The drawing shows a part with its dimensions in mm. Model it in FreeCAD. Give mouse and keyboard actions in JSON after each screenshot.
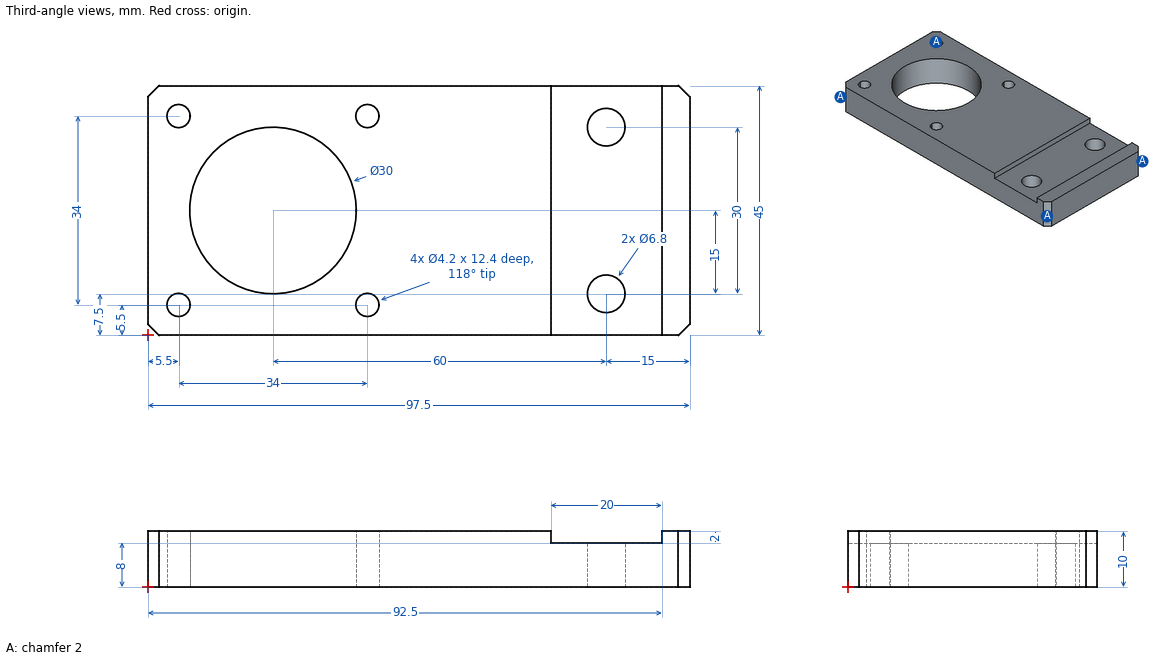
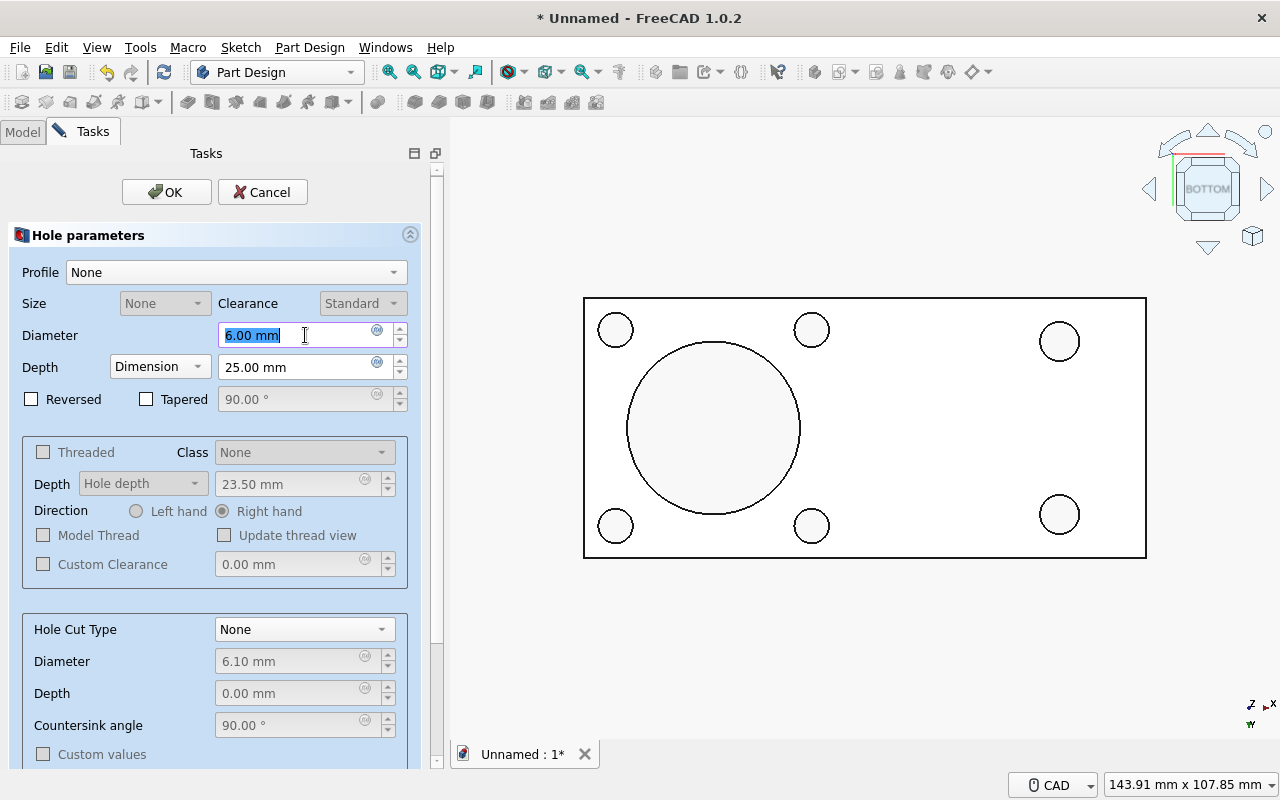
{"action": "type", "text": "4.2"}
{"action": "key", "text": "Tab"}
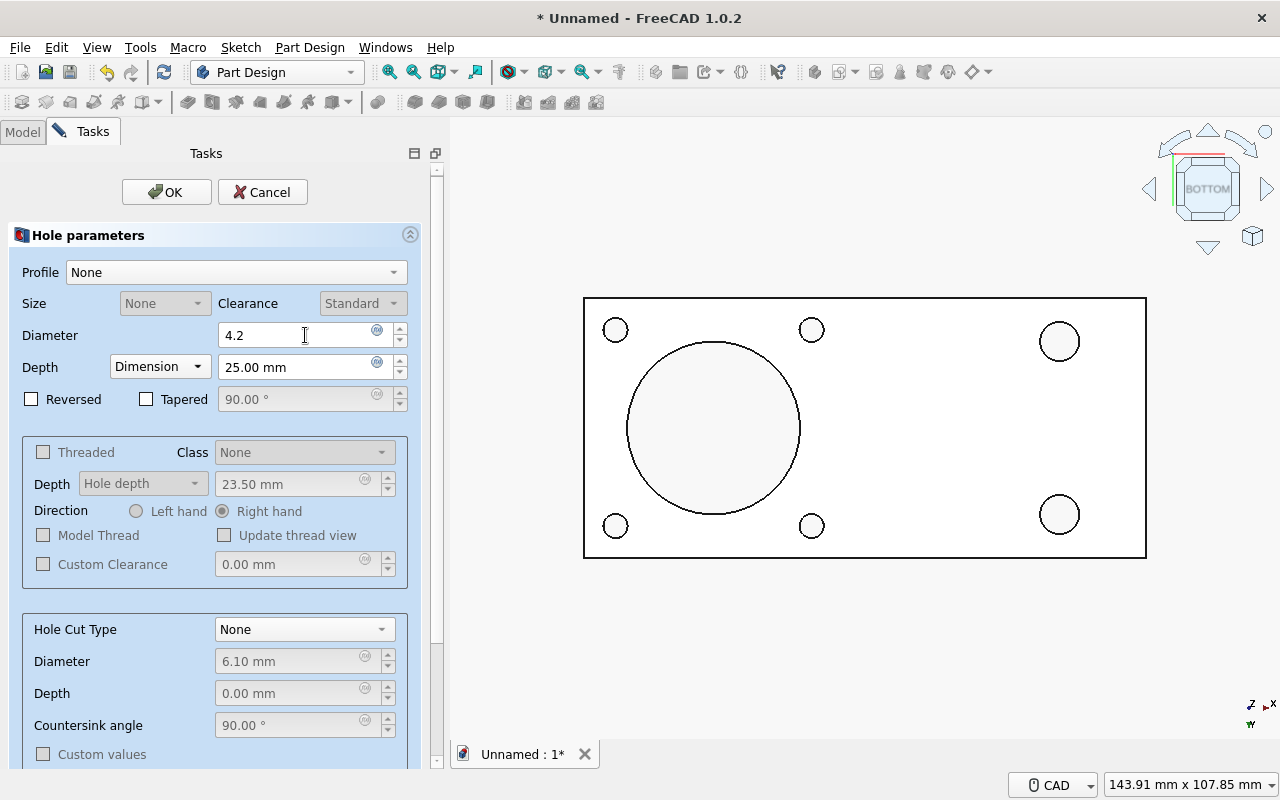
{"action": "triple_click", "coordinate": [305, 367]}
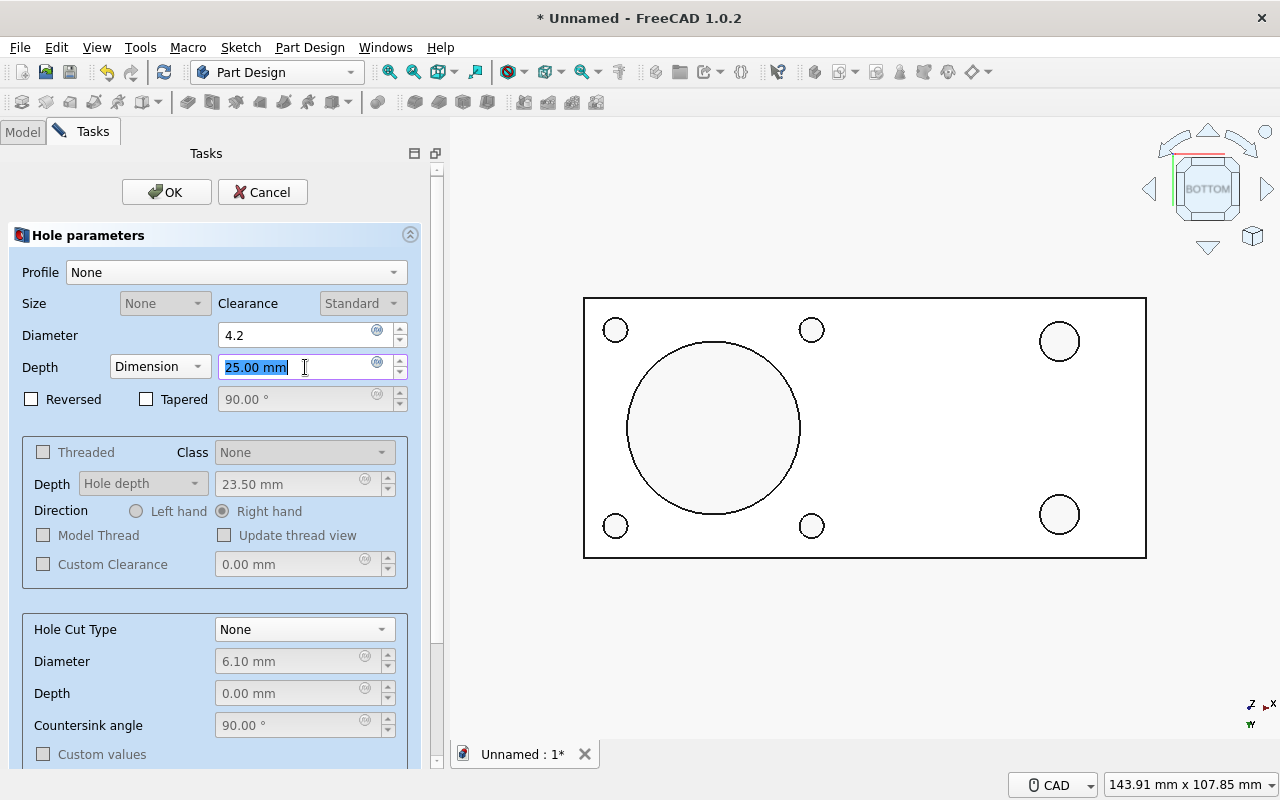
{"action": "type", "text": "12.4"}
{"action": "key", "text": "Tab"}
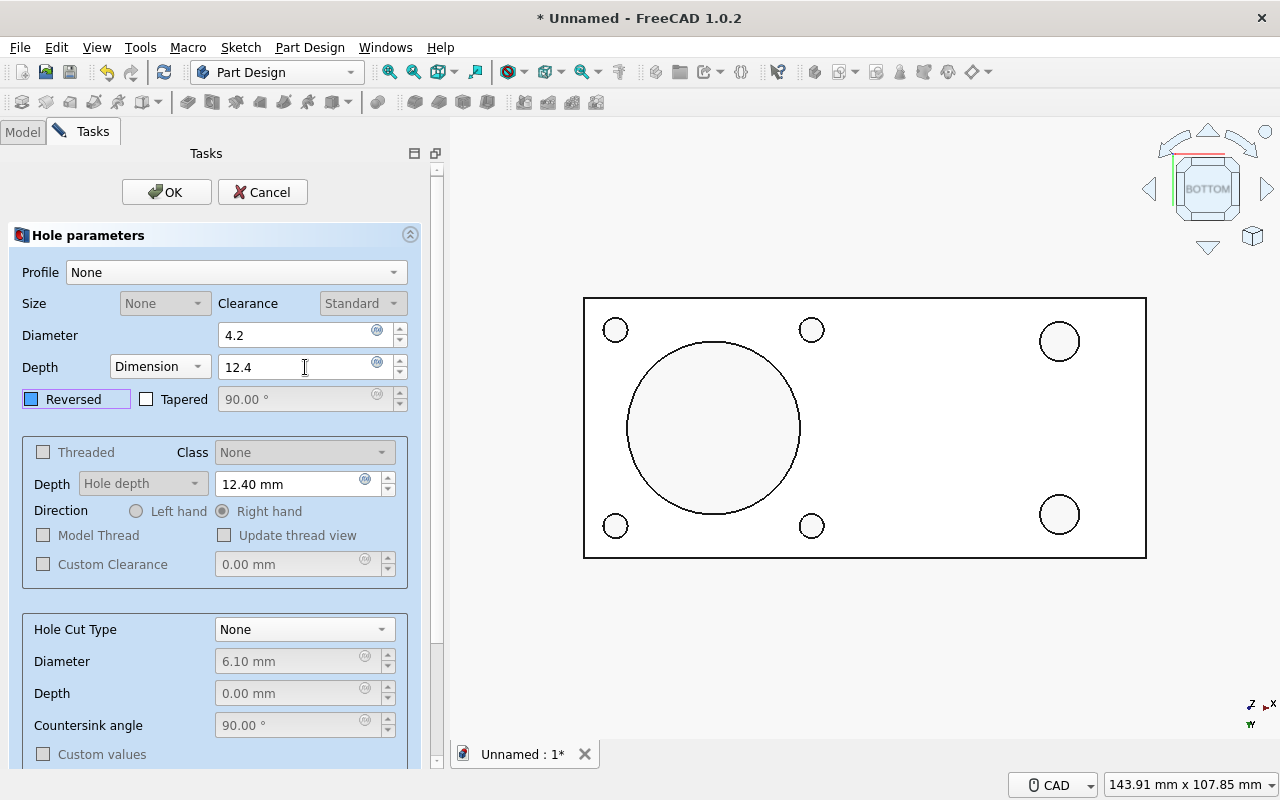
{"action": "left_click", "coordinate": [167, 192]}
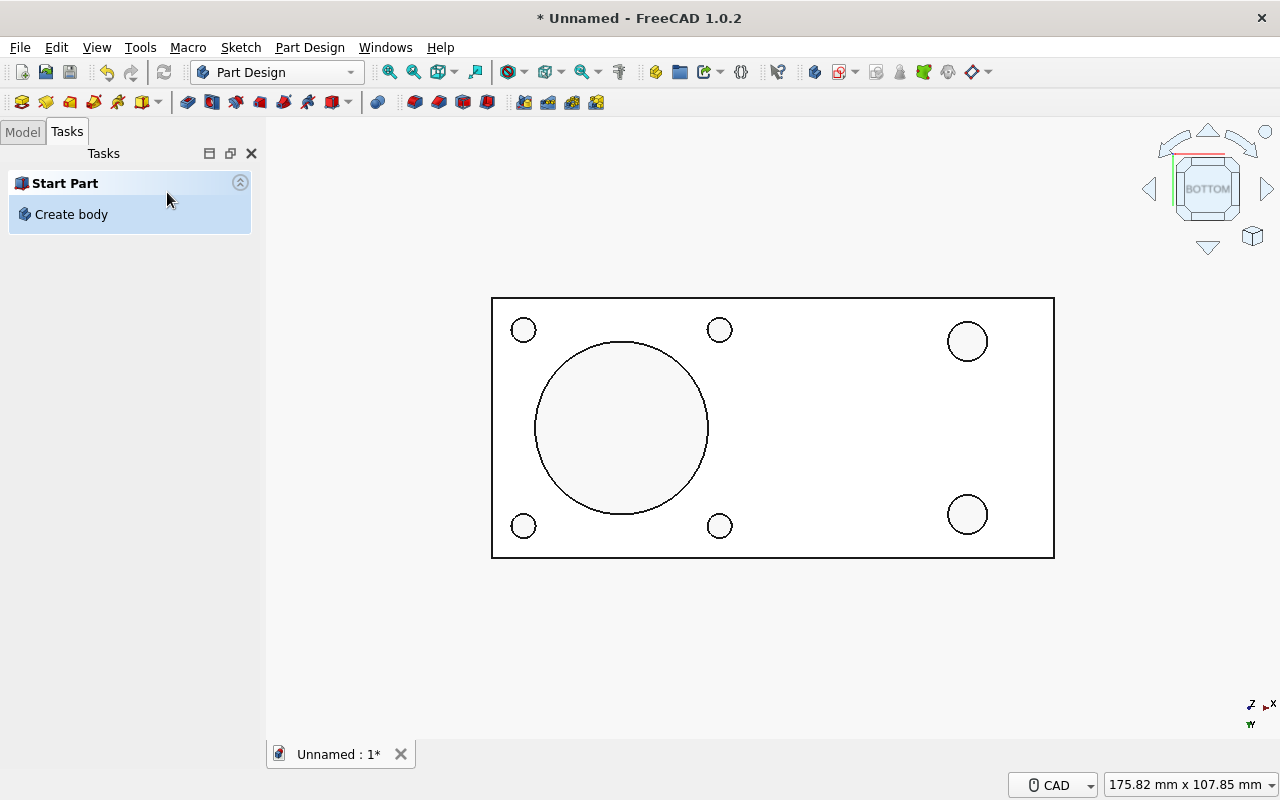
{"action": "key", "text": "0"}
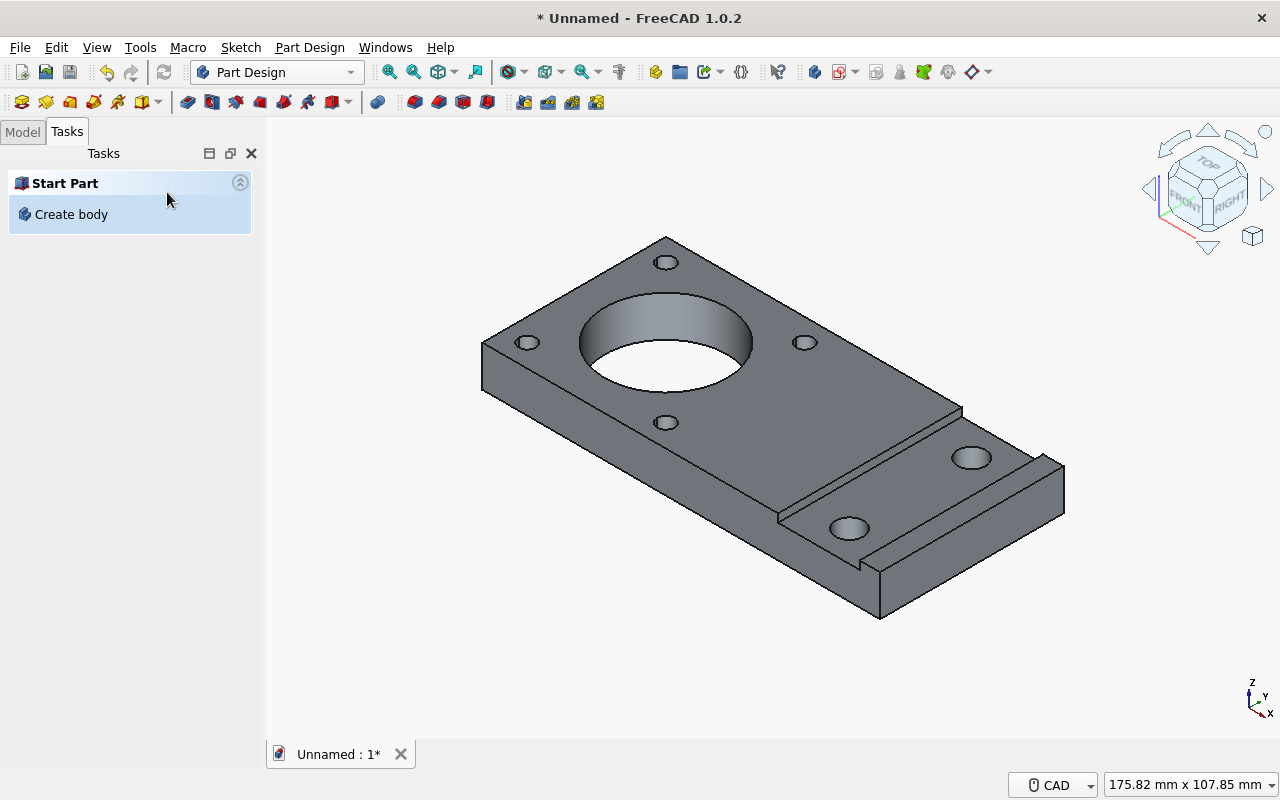
{"action": "left_click", "coordinate": [880, 595]}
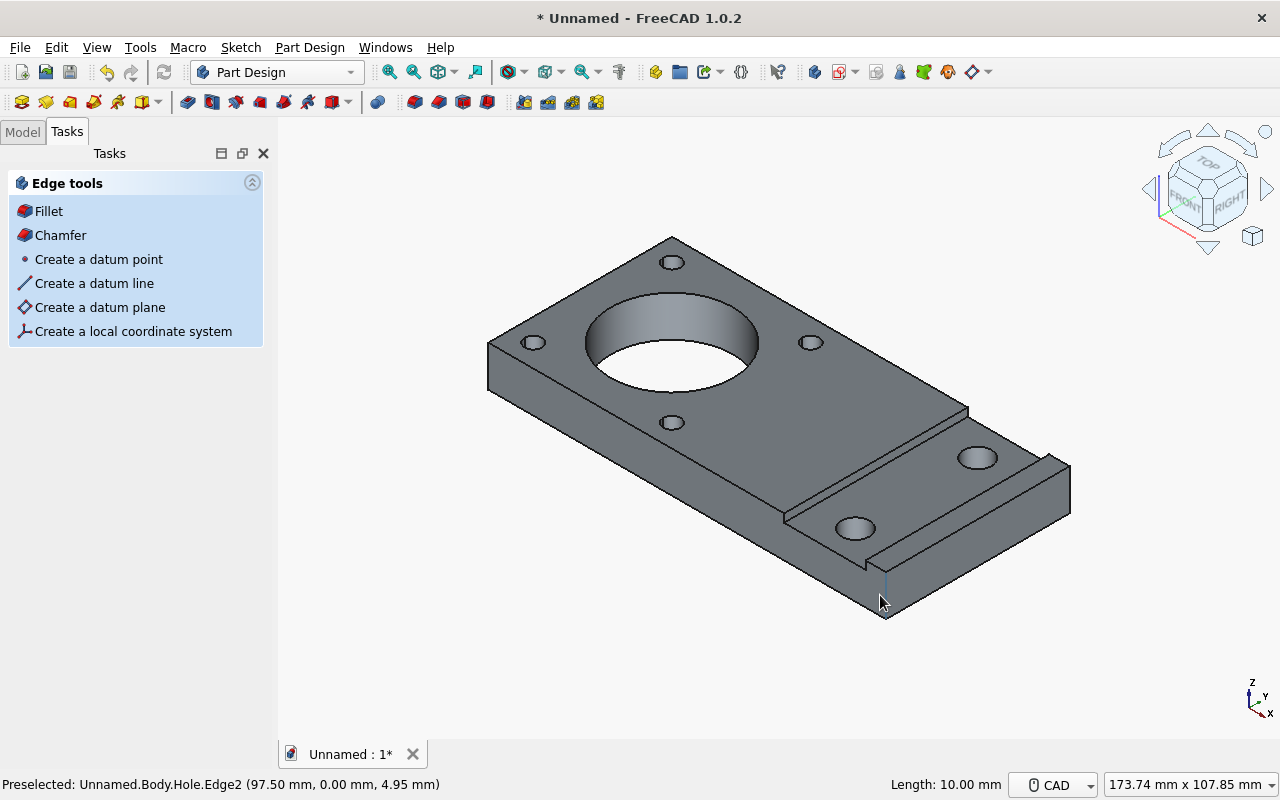
{"action": "key", "text": "2"}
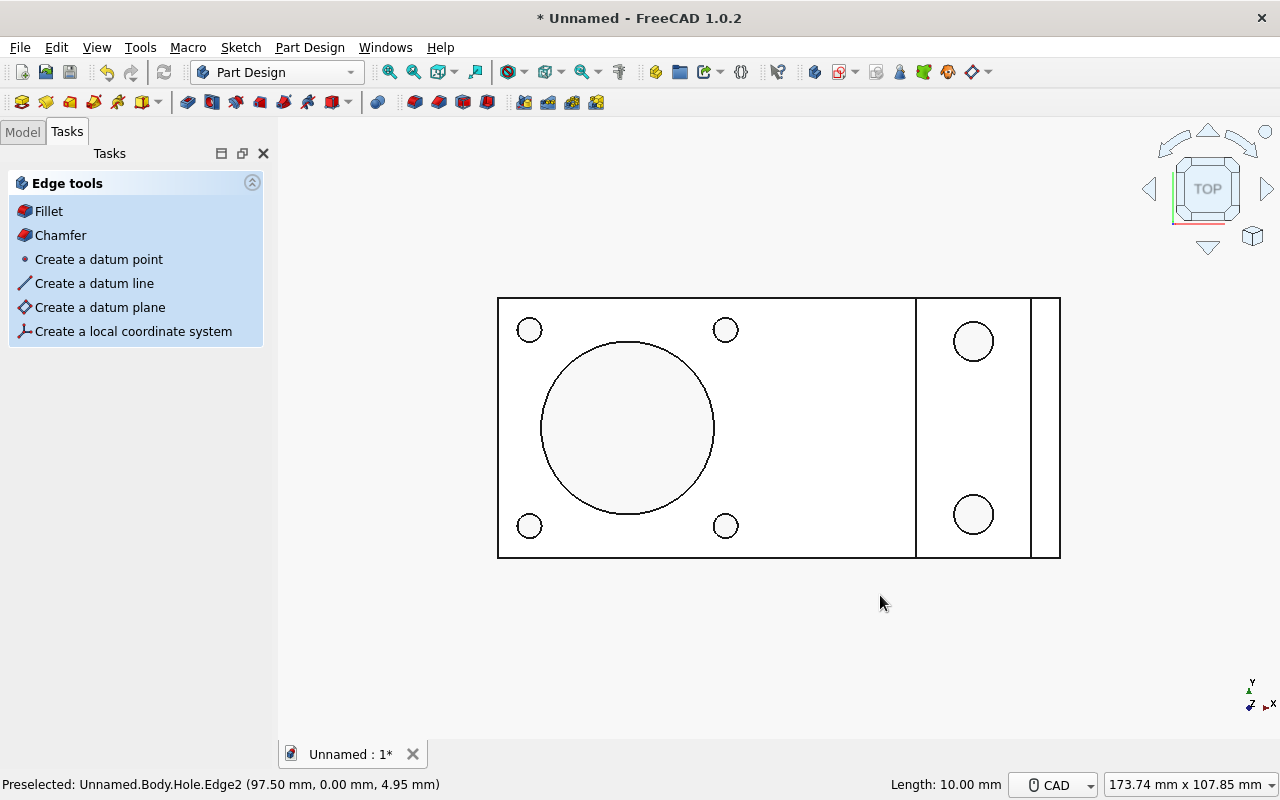
{"action": "key", "text": "1"}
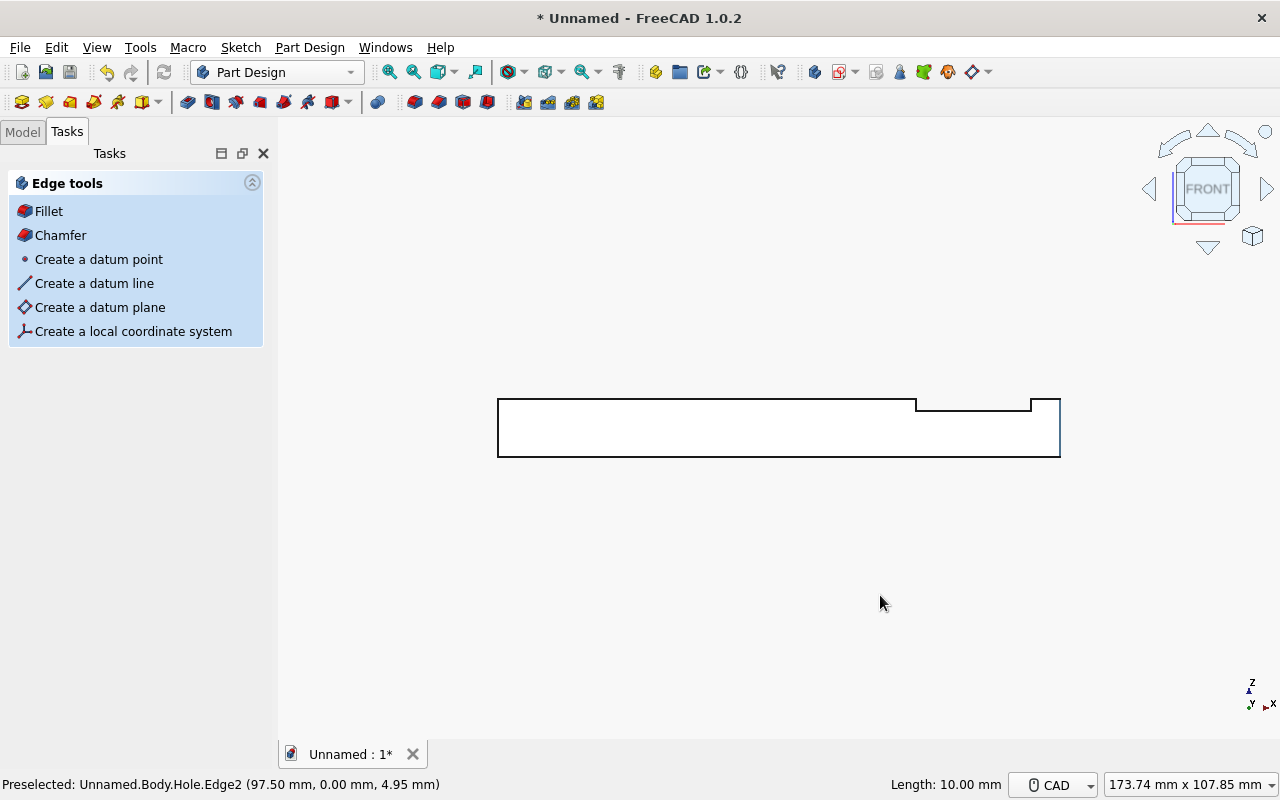
{"action": "left_click", "coordinate": [498, 427], "text": "ctrl"}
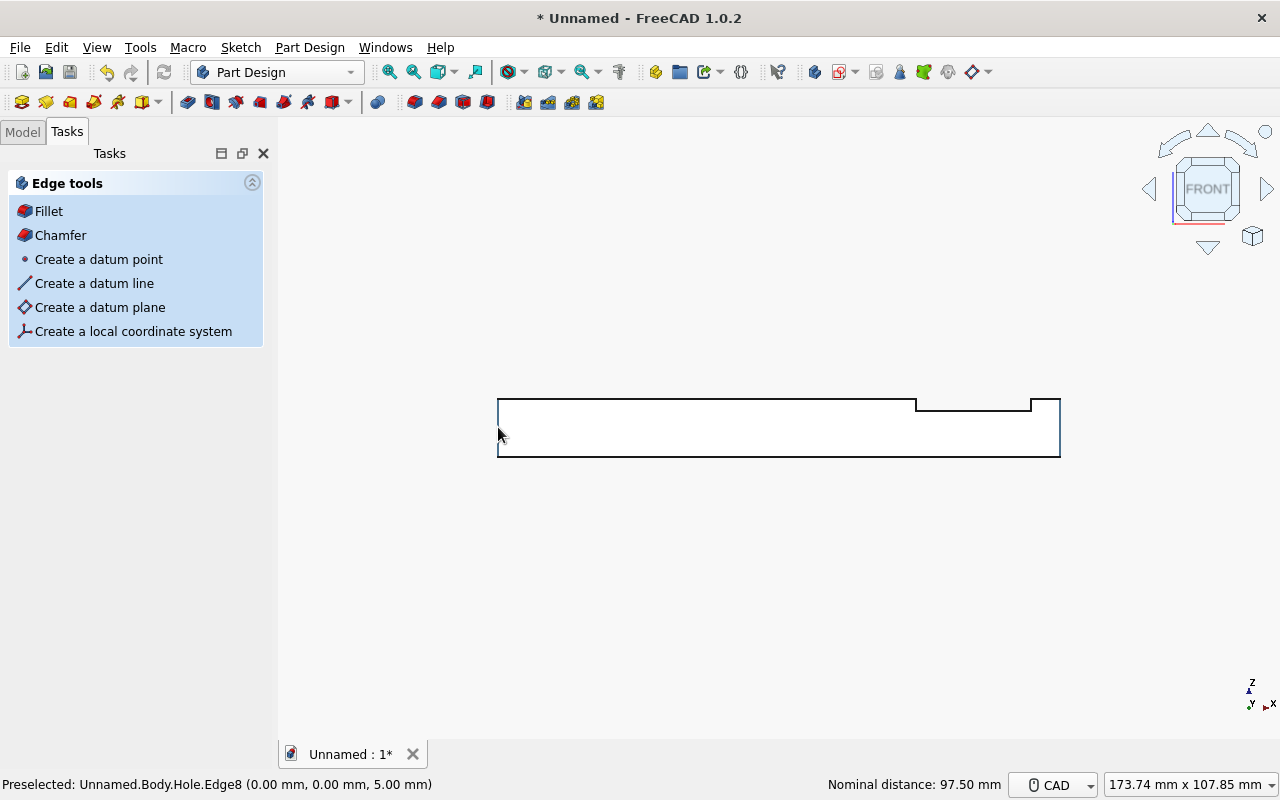
{"action": "key", "text": "3"}